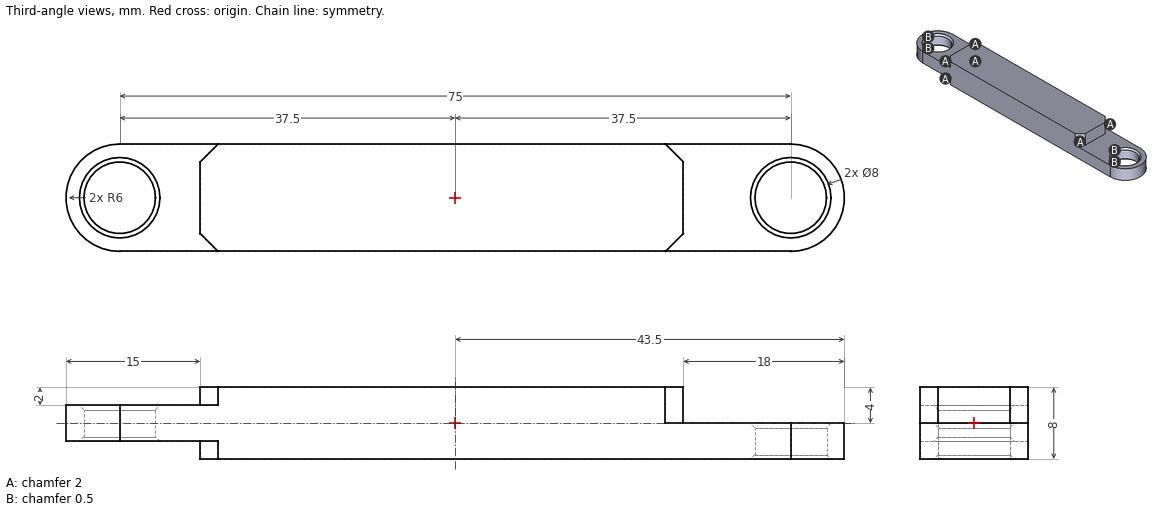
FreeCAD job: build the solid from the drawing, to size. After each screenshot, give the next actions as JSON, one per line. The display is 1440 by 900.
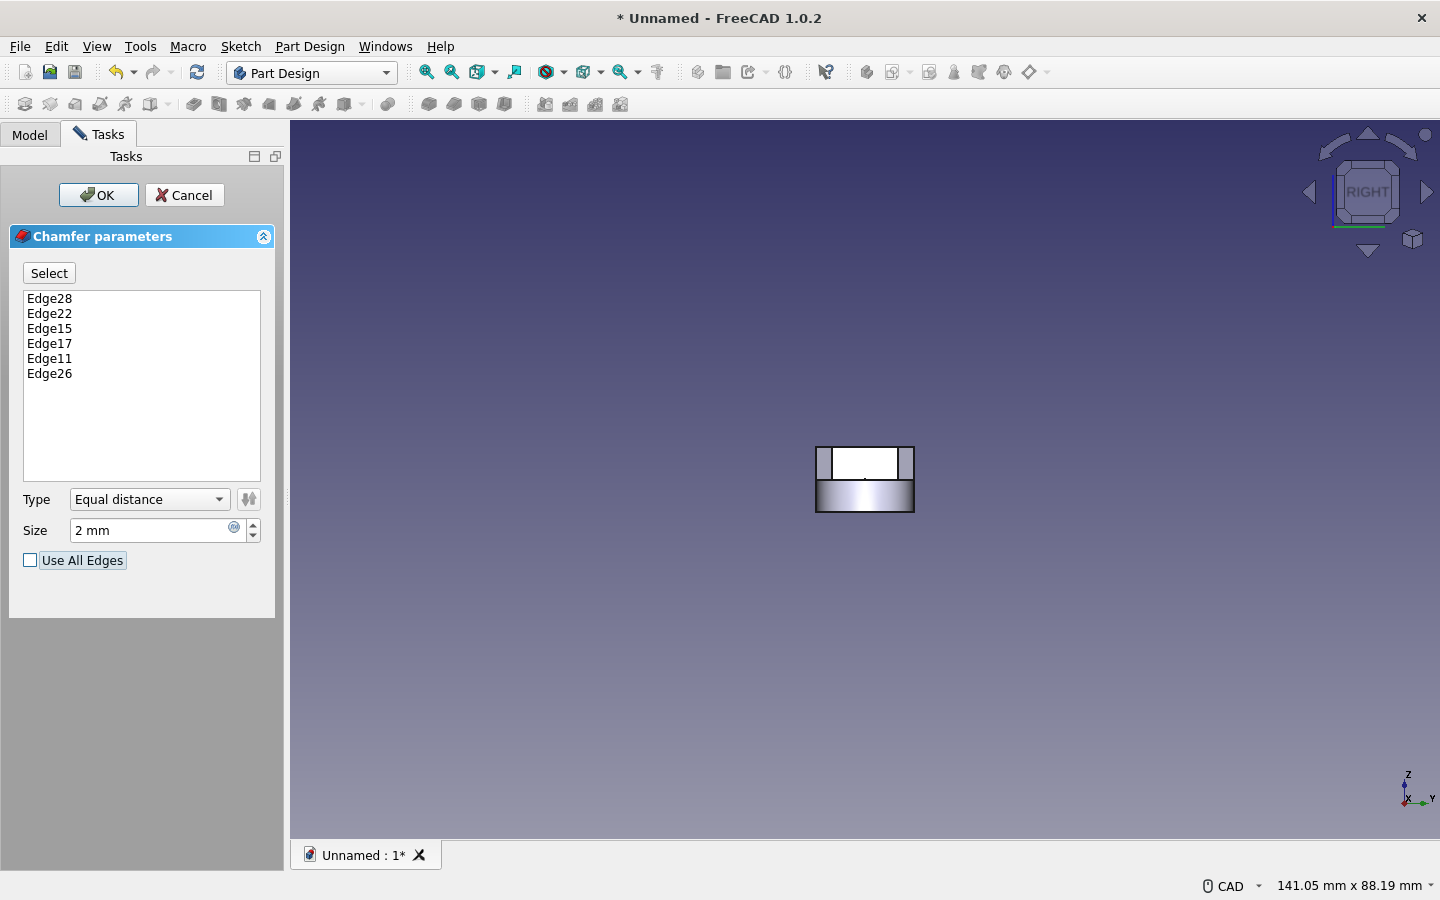
{"action": "left_click", "coordinate": [99, 195]}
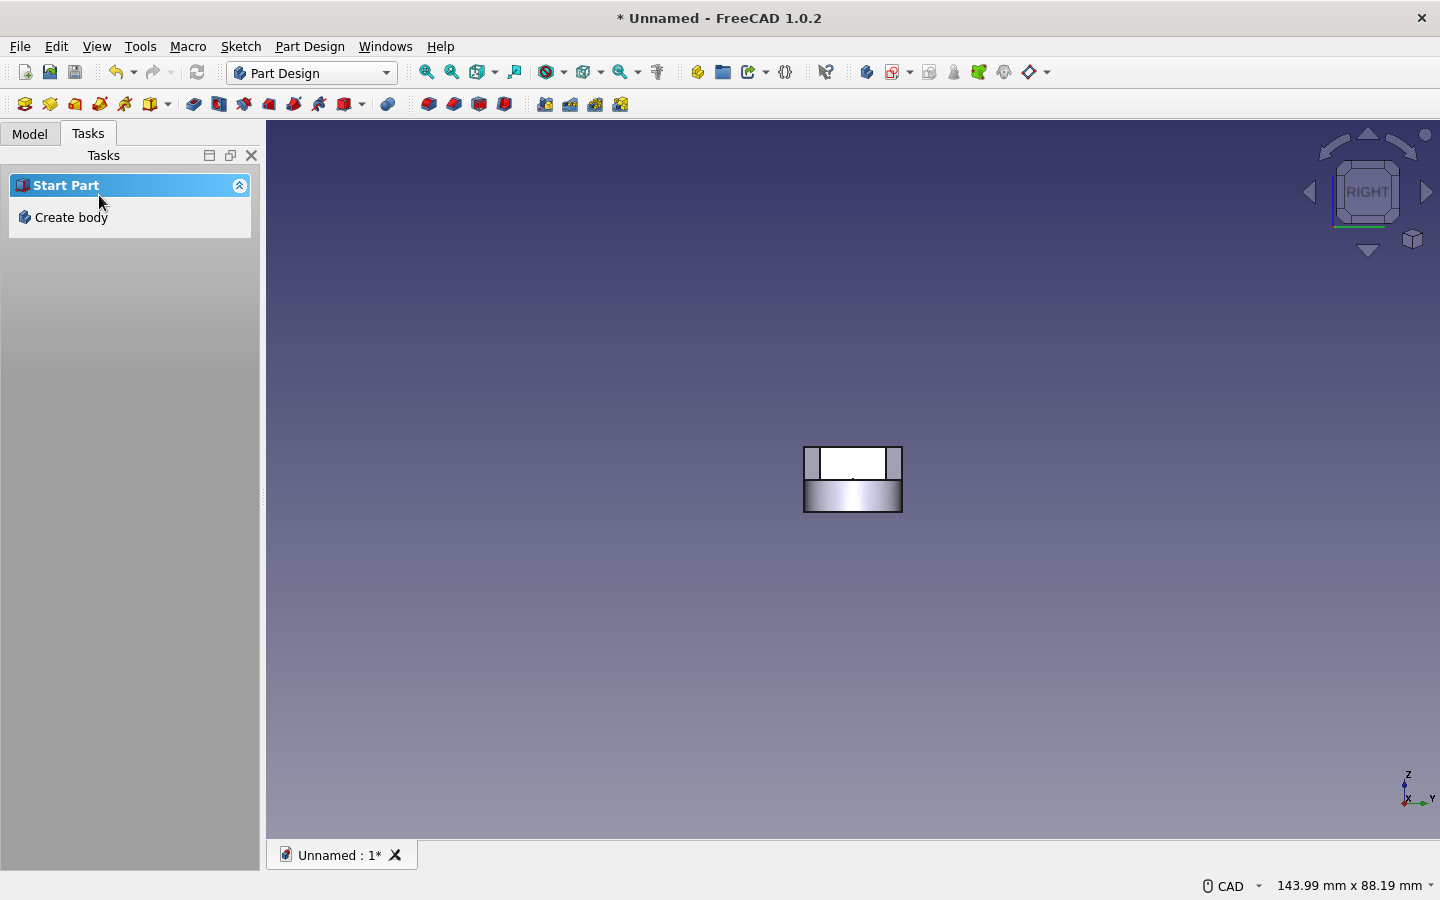
{"action": "left_click", "coordinate": [427, 72]}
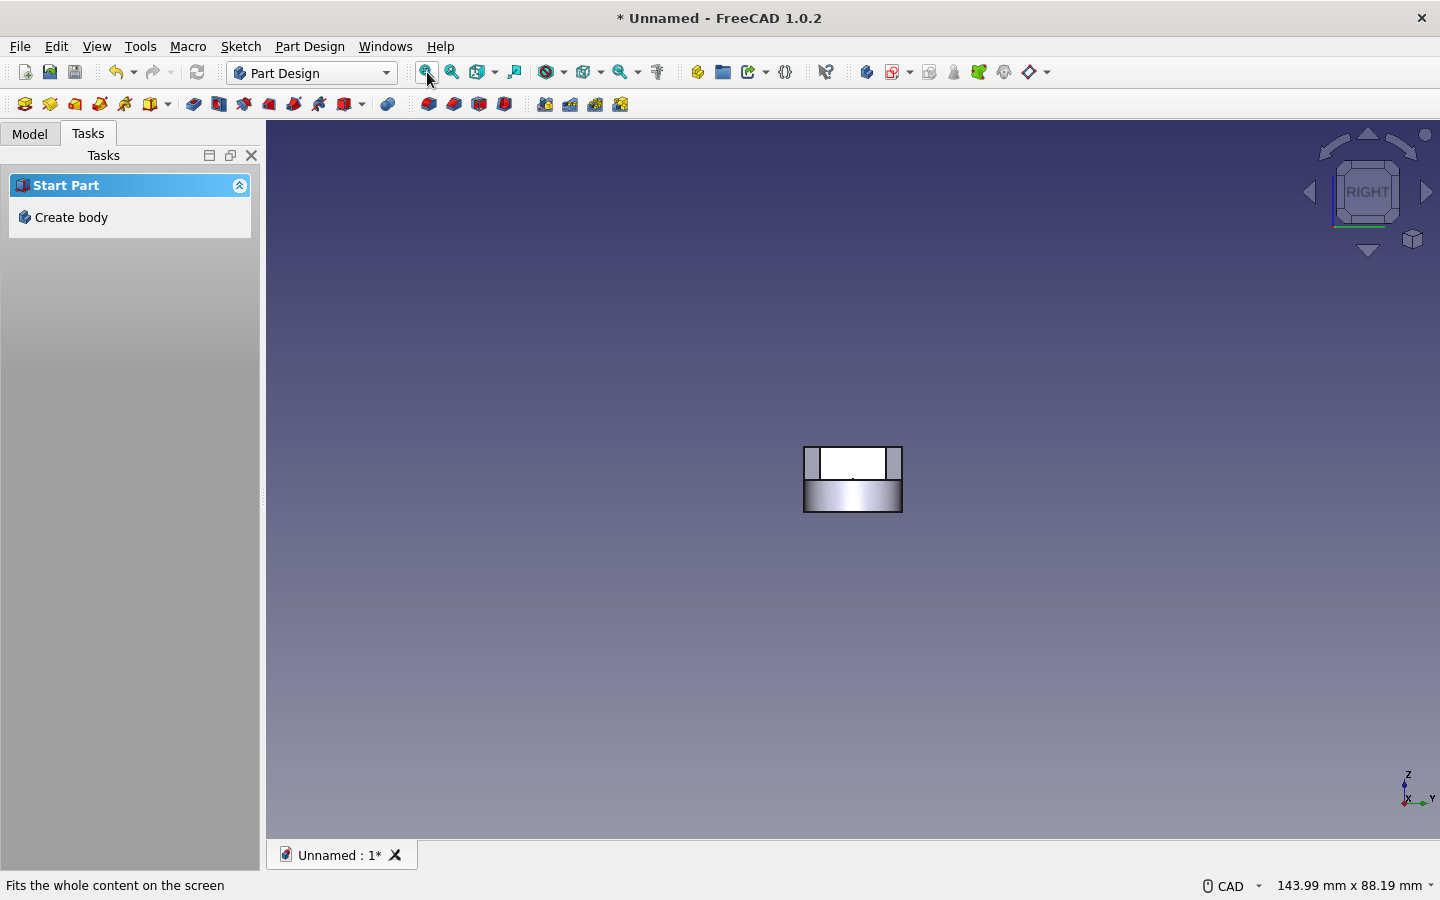
{"action": "key", "text": "0"}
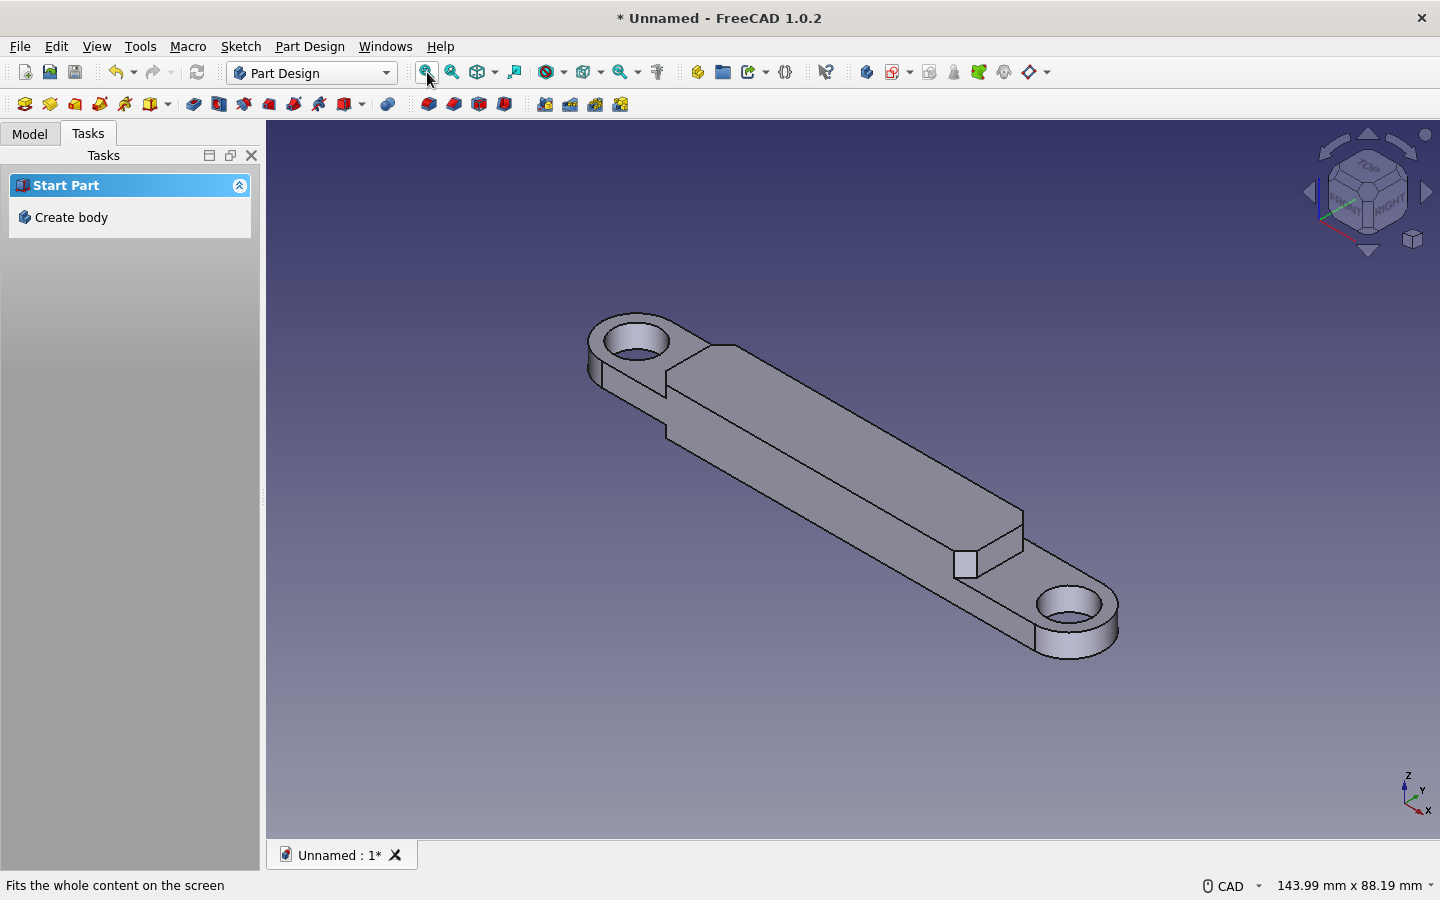
{"action": "left_click", "coordinate": [1046, 590]}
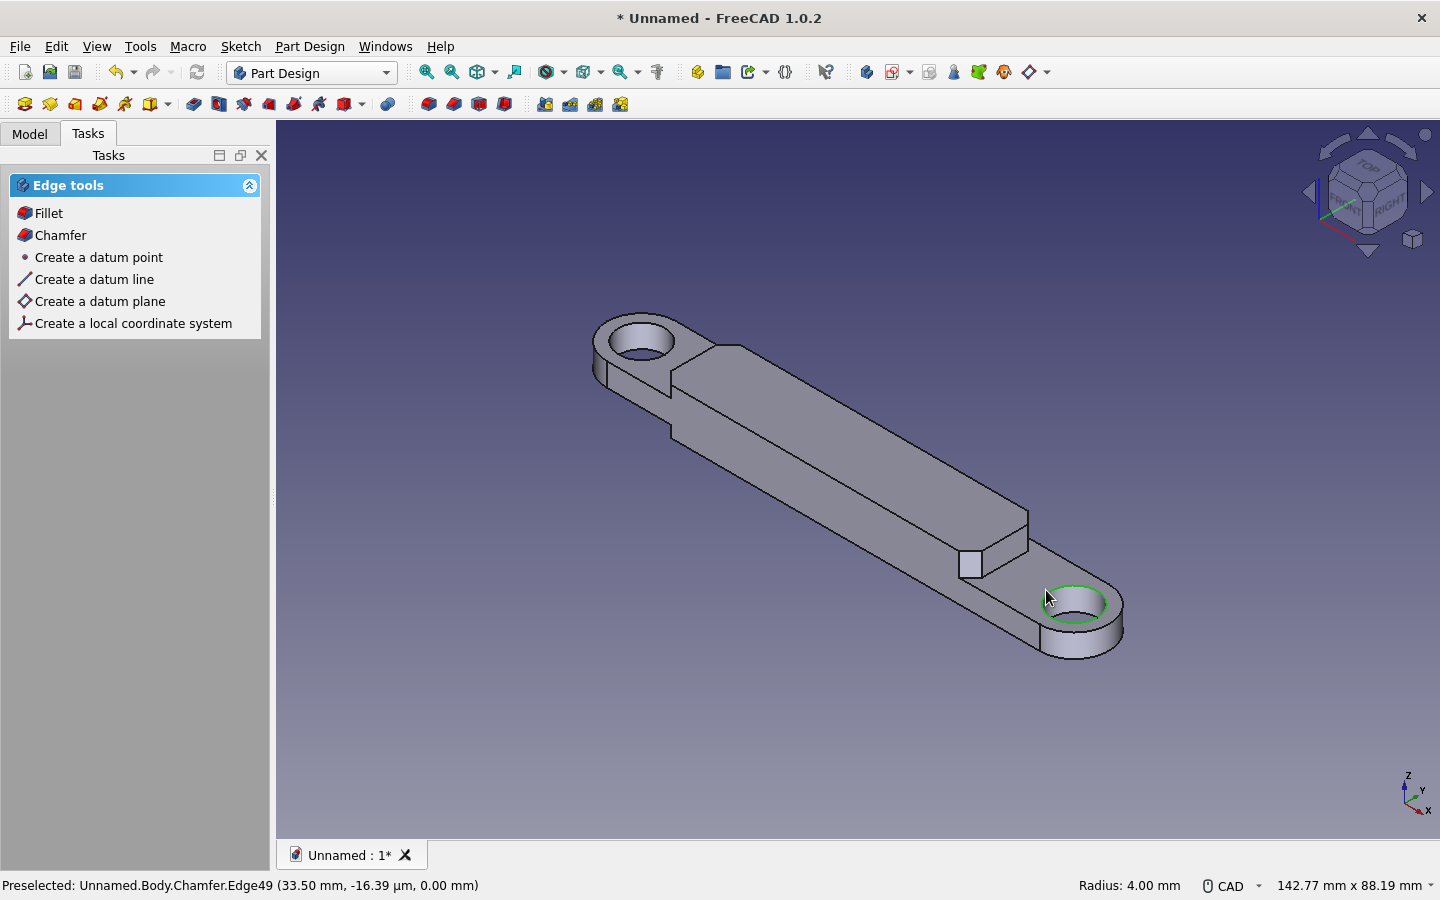
{"action": "left_click", "coordinate": [619, 327], "text": "ctrl"}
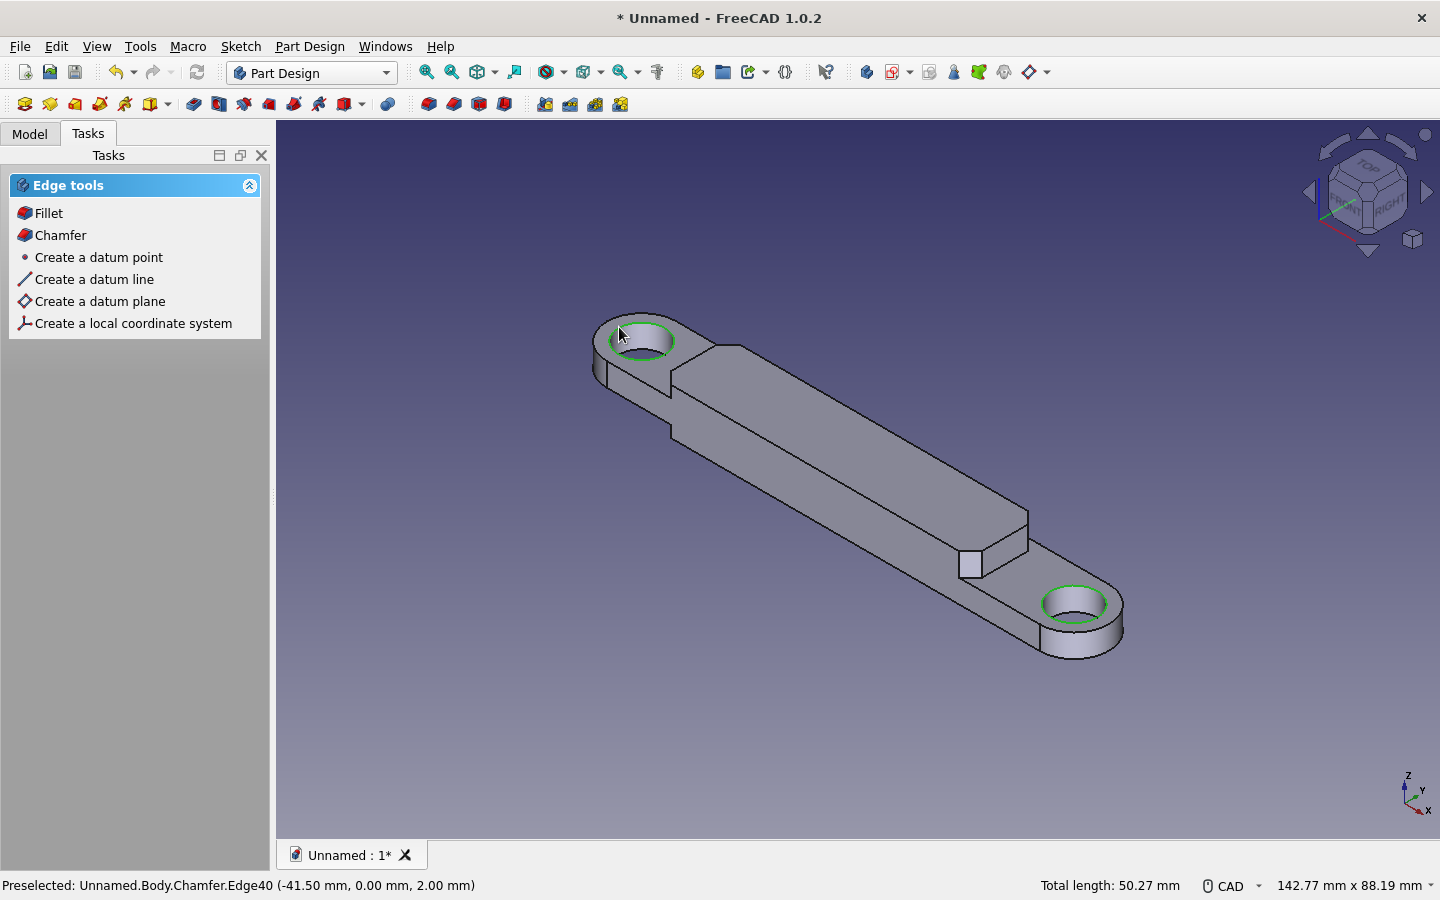
{"action": "key", "text": "2"}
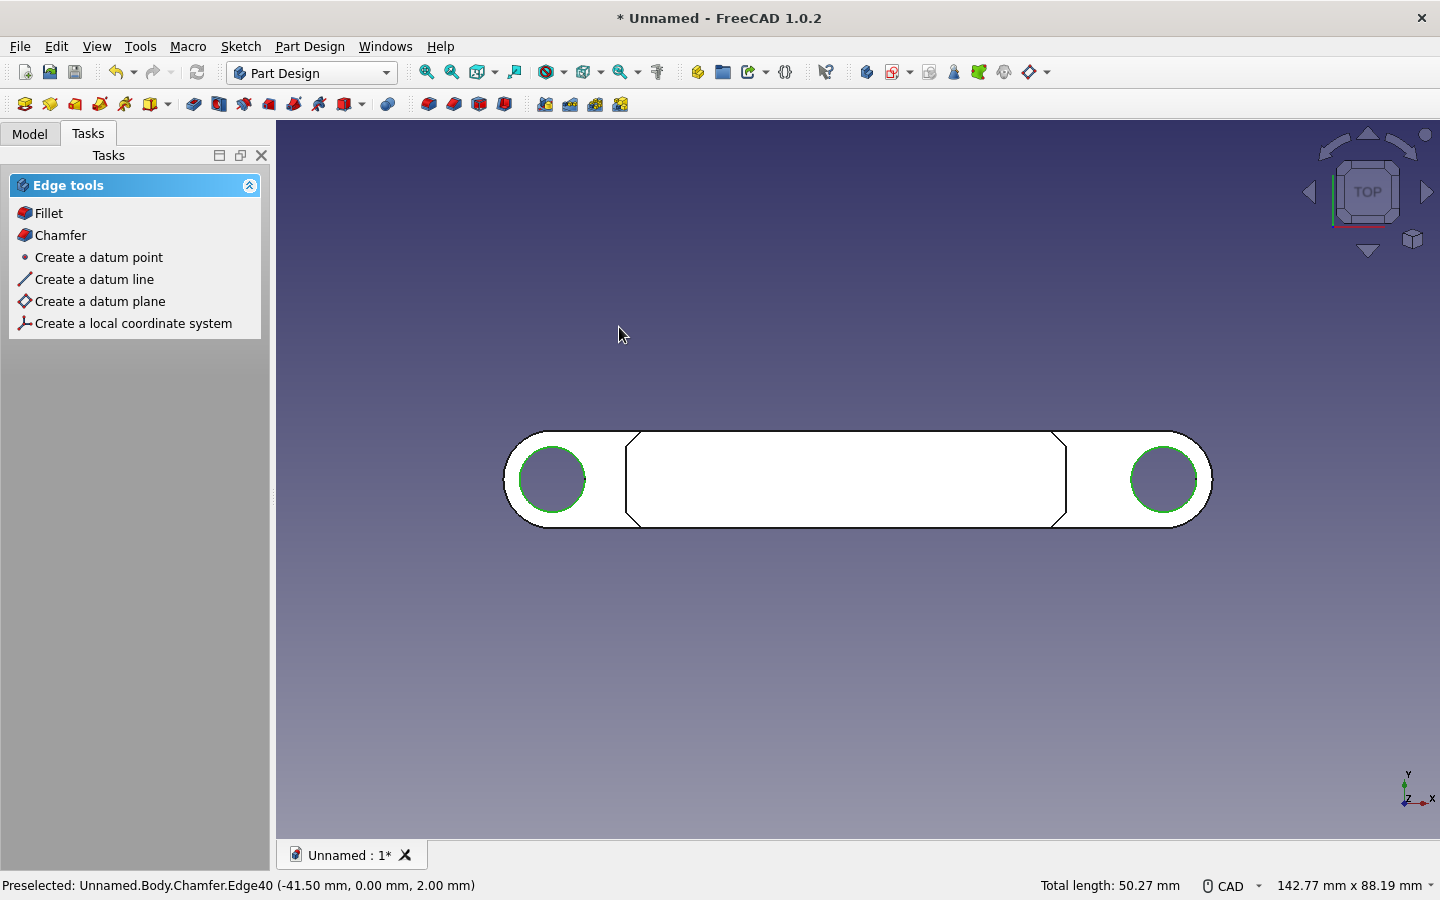
{"action": "key", "text": "1"}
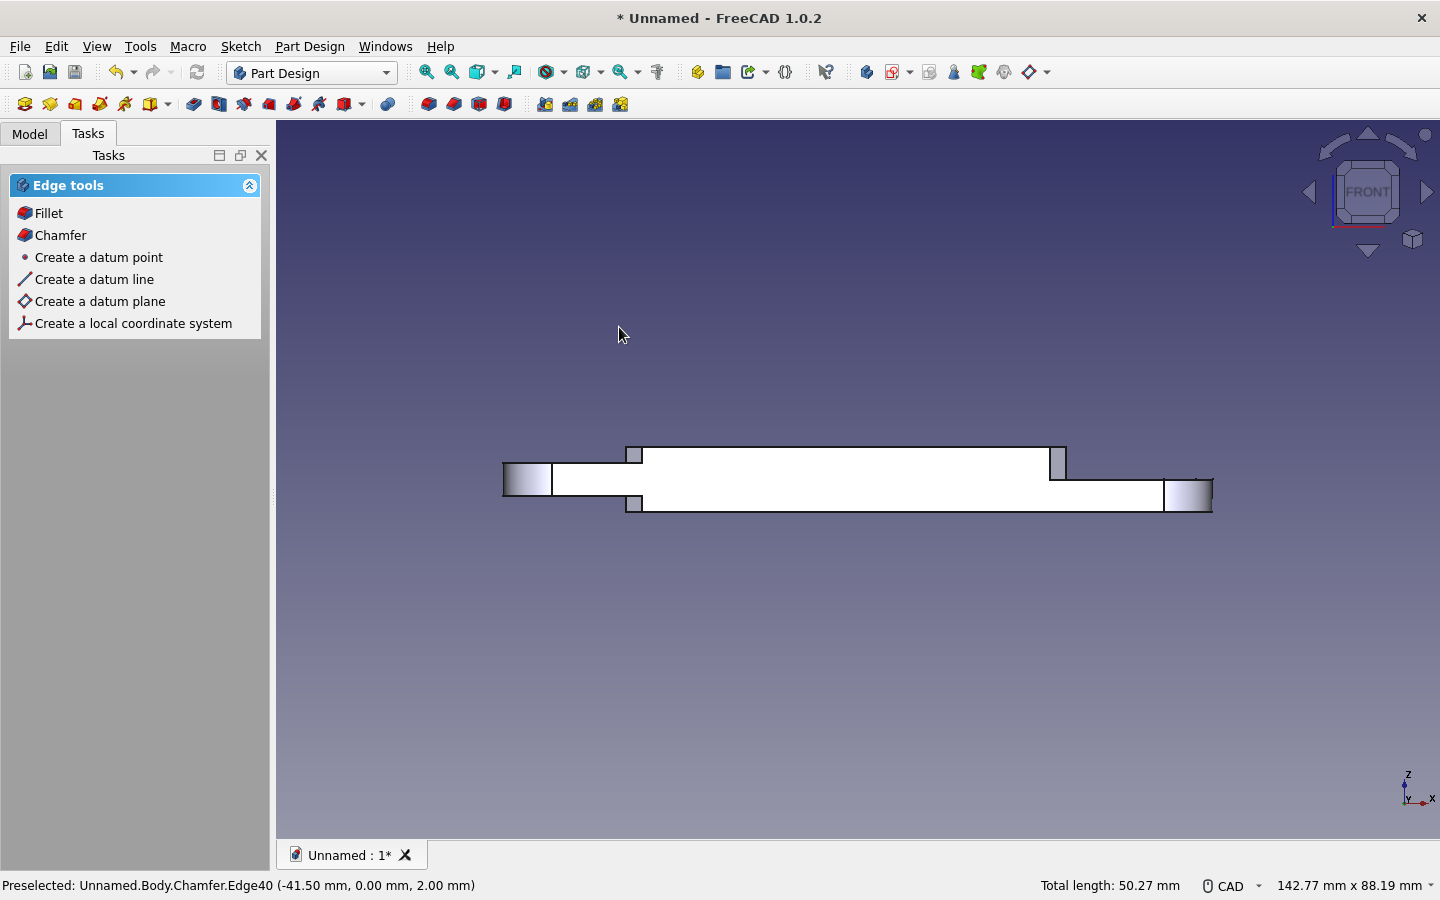
{"action": "key", "text": "3"}